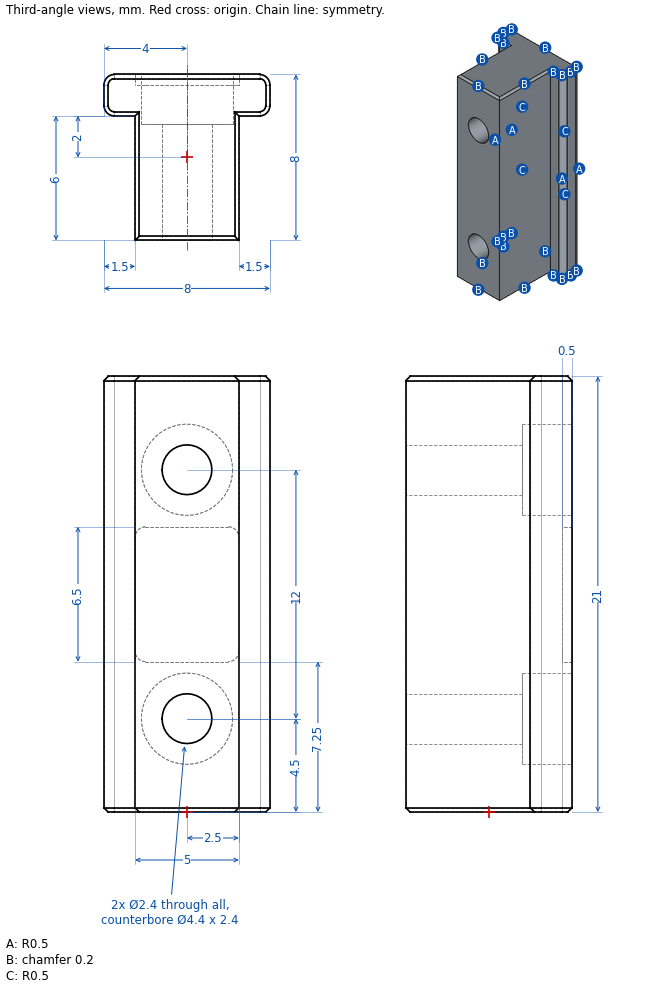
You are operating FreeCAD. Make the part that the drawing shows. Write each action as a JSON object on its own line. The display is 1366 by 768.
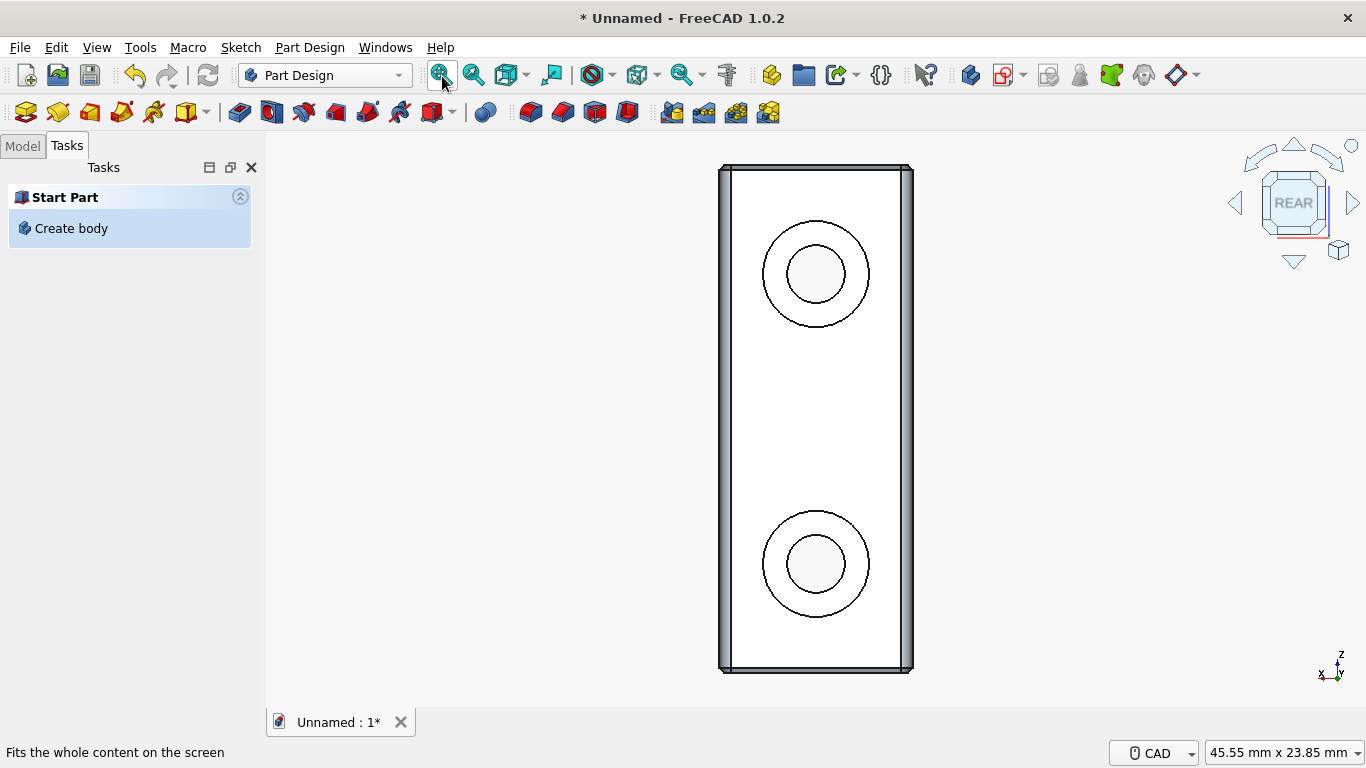
{"action": "left_click", "coordinate": [816, 418]}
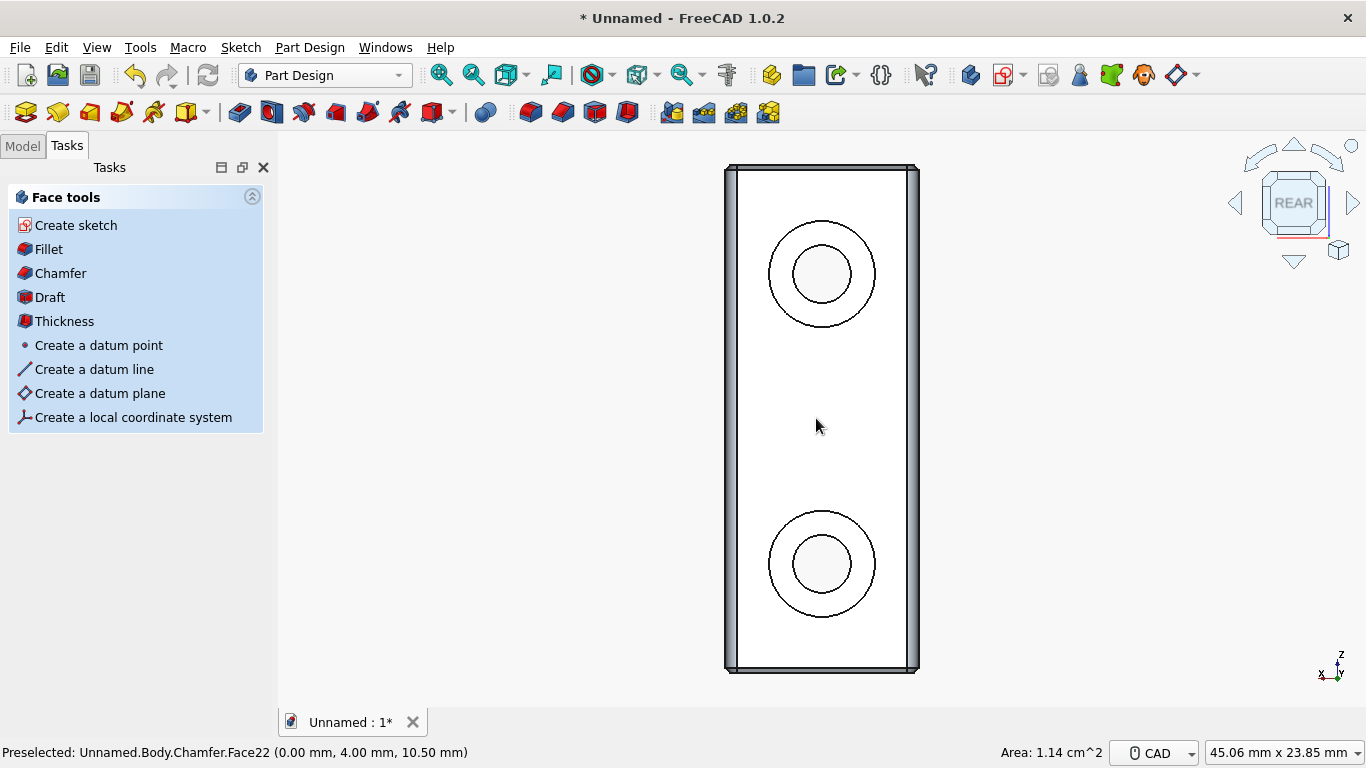
{"action": "left_click", "coordinate": [1004, 76]}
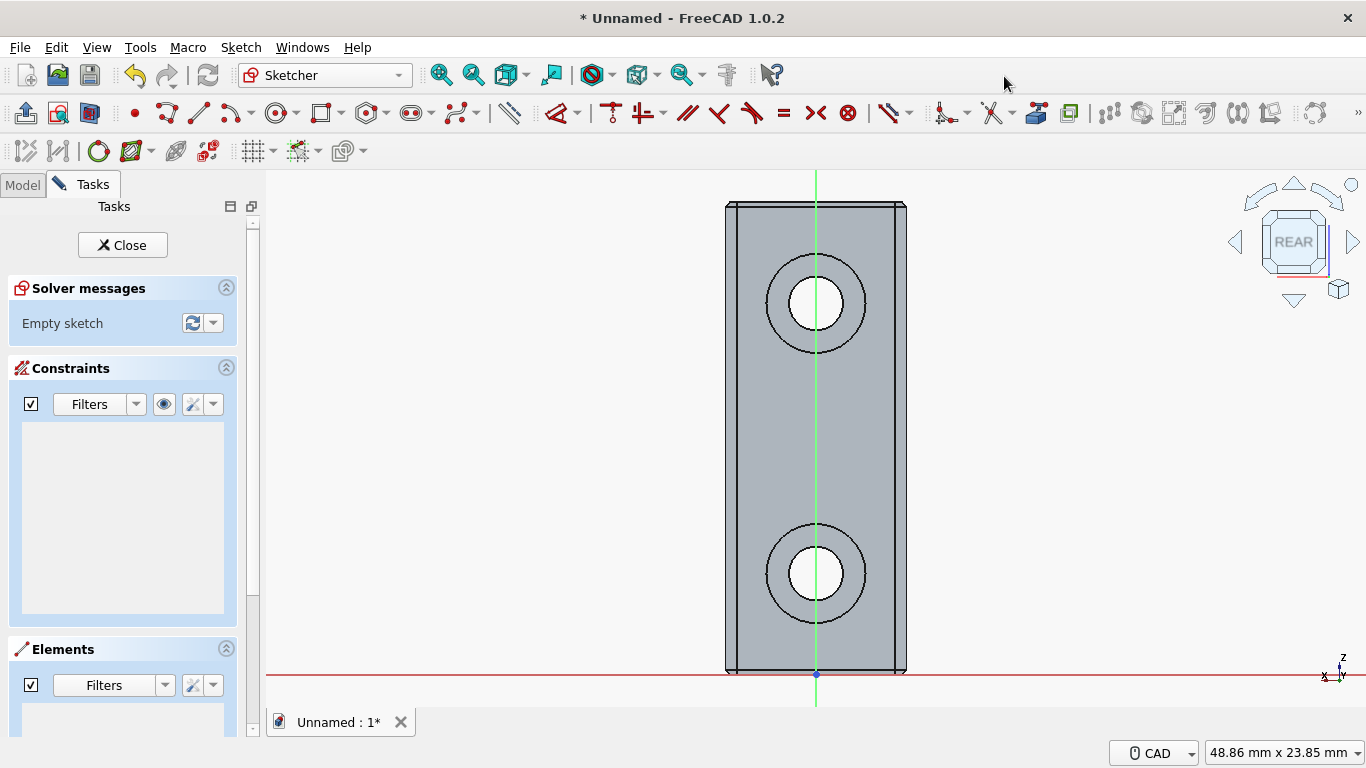
{"action": "scroll", "coordinate": [438, 198], "scroll_direction": "down", "scroll_amount": 1}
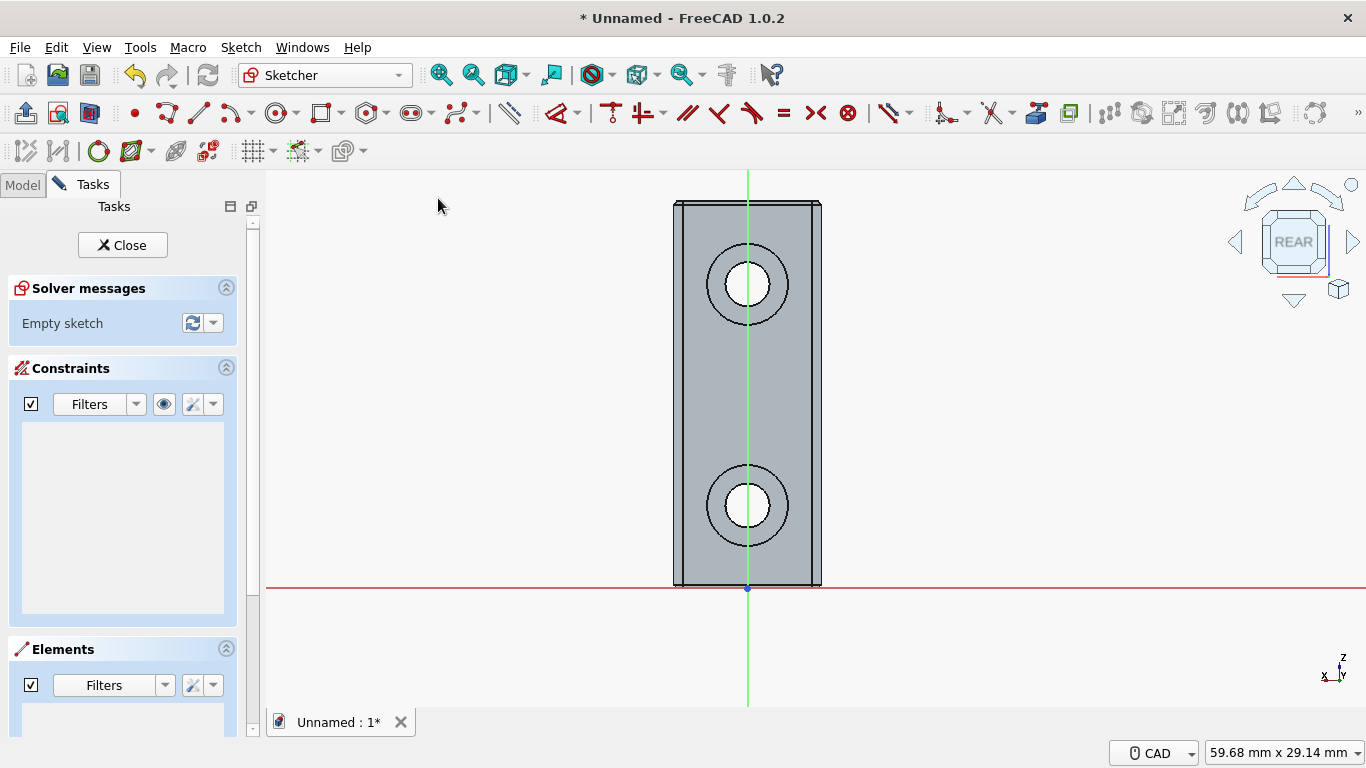
{"action": "left_click", "coordinate": [322, 114]}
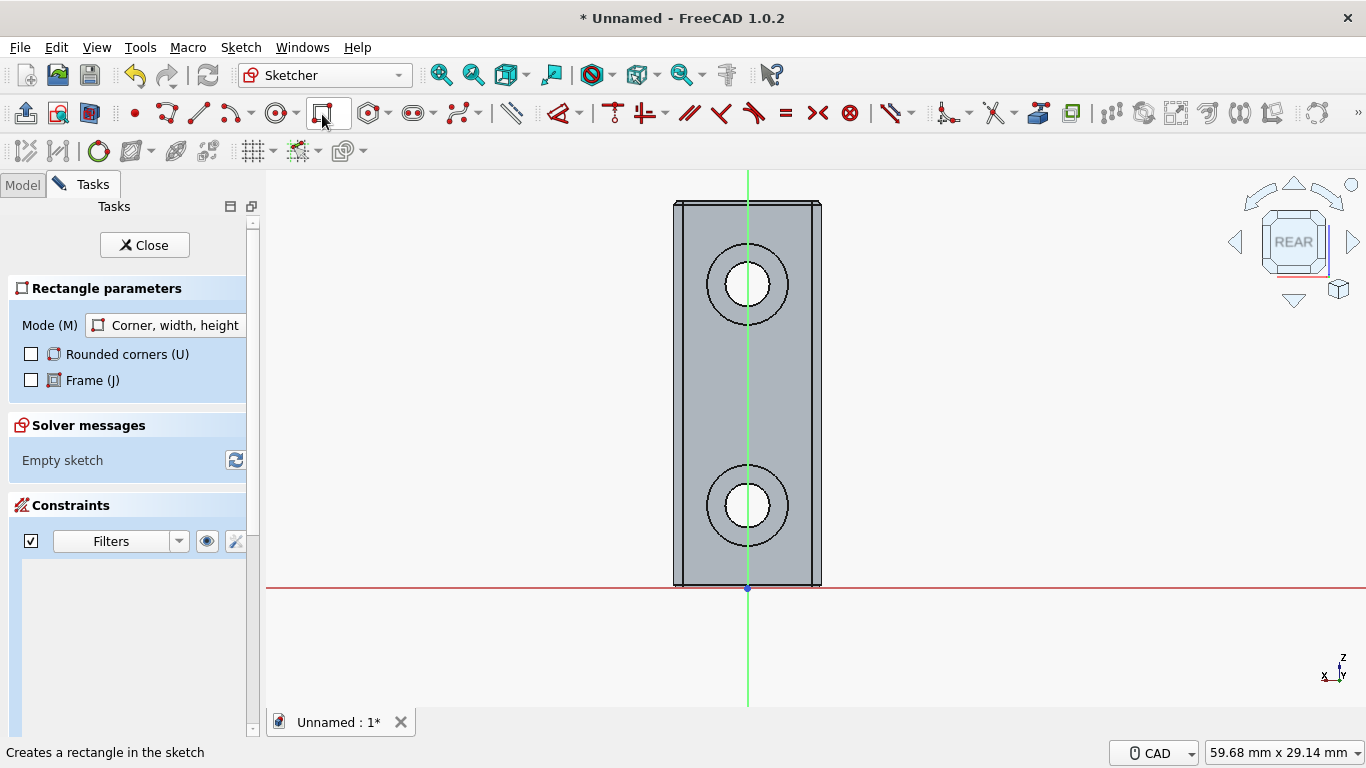
{"action": "left_click", "coordinate": [701, 335]}
{"action": "mouse_move", "coordinate": [794, 455]}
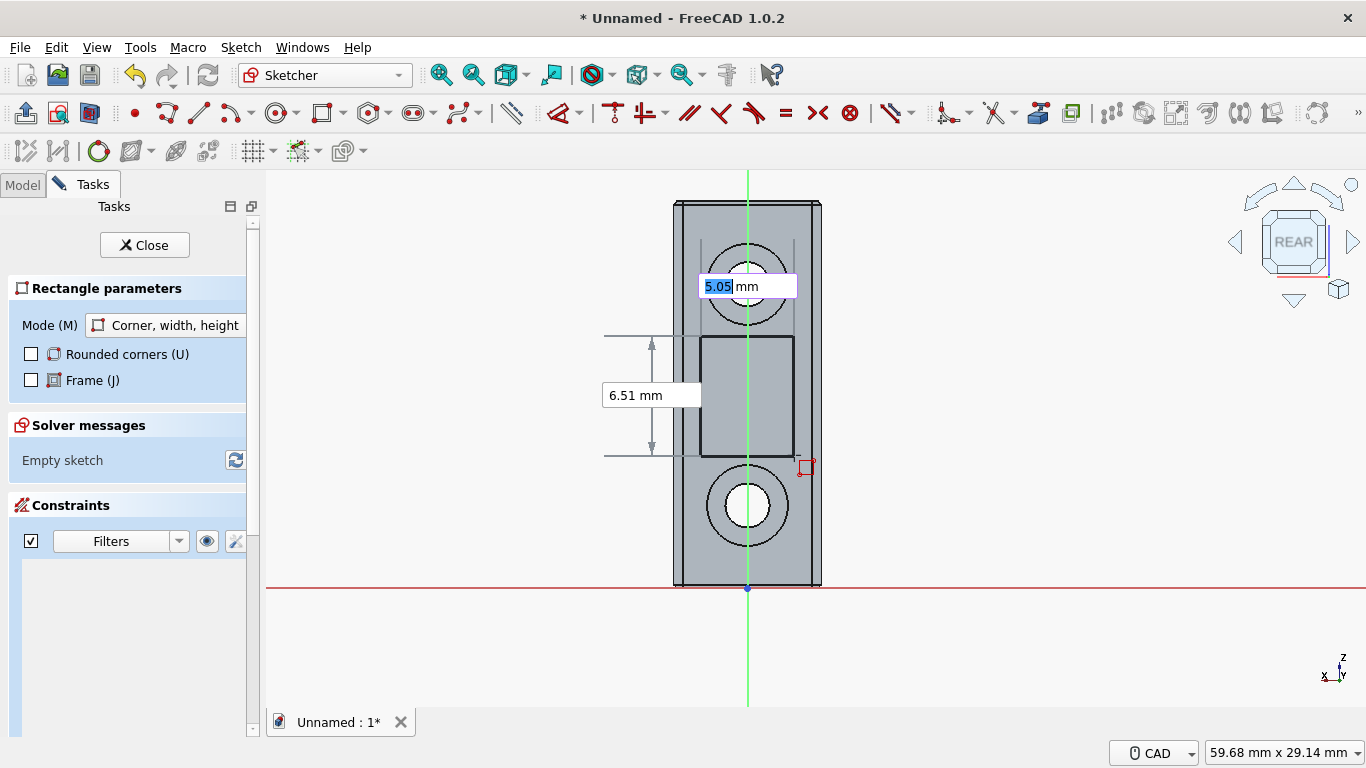
{"action": "type", "text": "5"}
{"action": "key", "text": "Tab"}
{"action": "type", "text": "6.5"}
{"action": "key", "text": "Return"}
{"action": "key", "text": "Escape"}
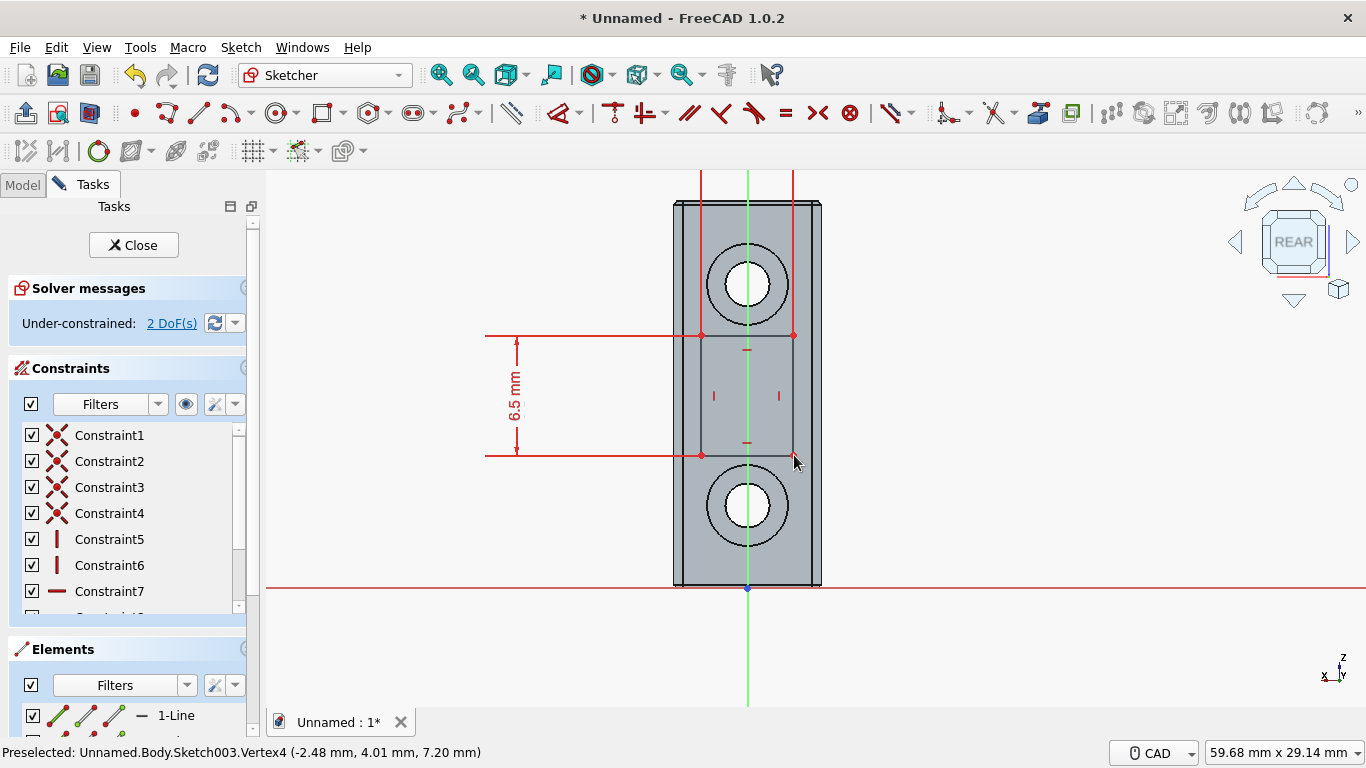
{"action": "left_click", "coordinate": [558, 114]}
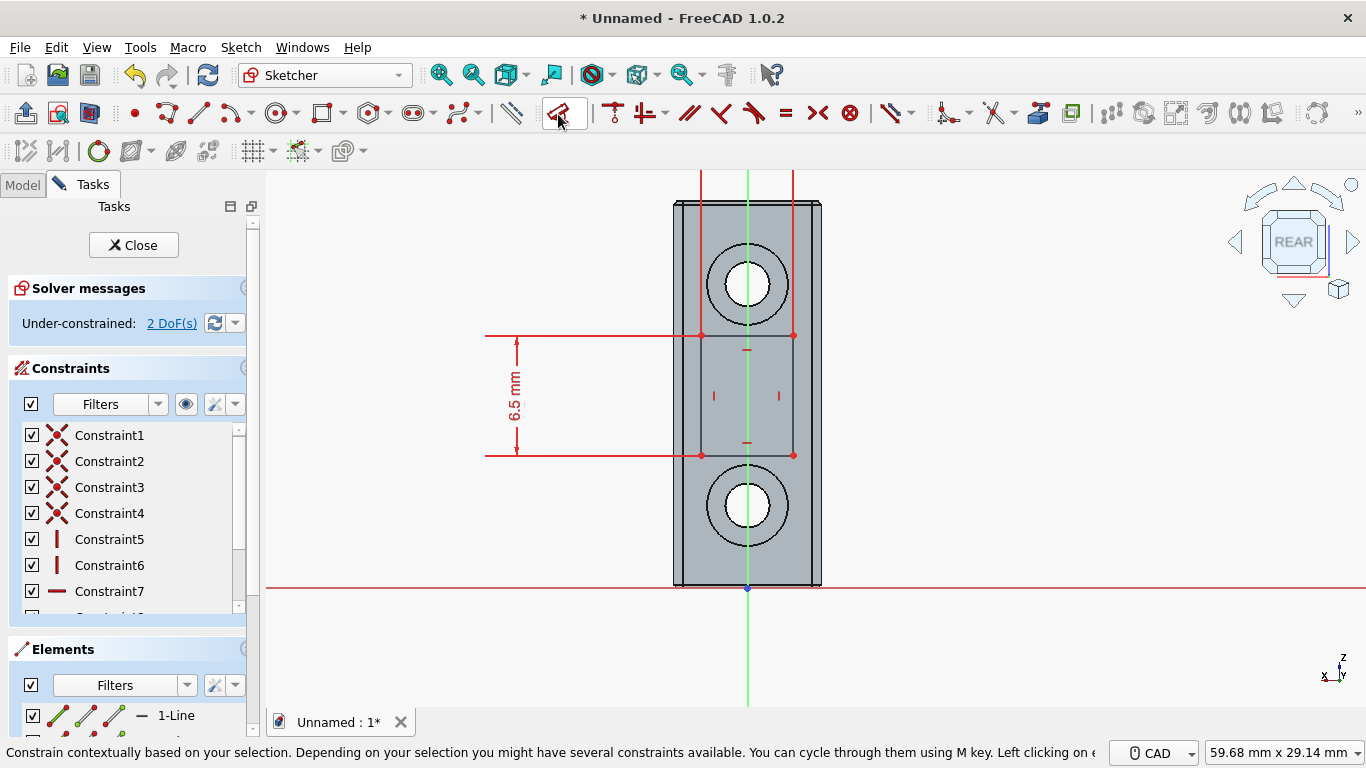
{"action": "left_click", "coordinate": [701, 336]}
{"action": "left_click", "coordinate": [724, 622]}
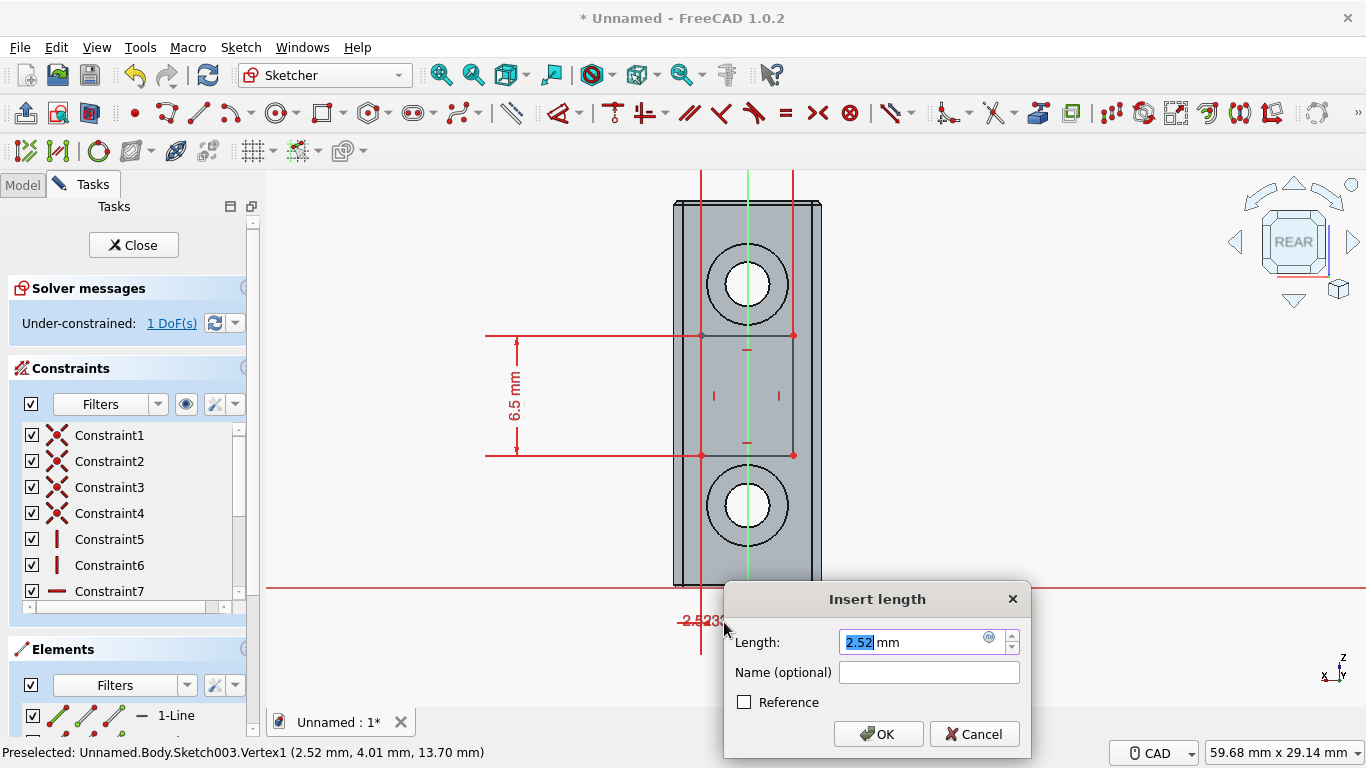
{"action": "type", "text": "2.5"}
{"action": "key", "text": "Return"}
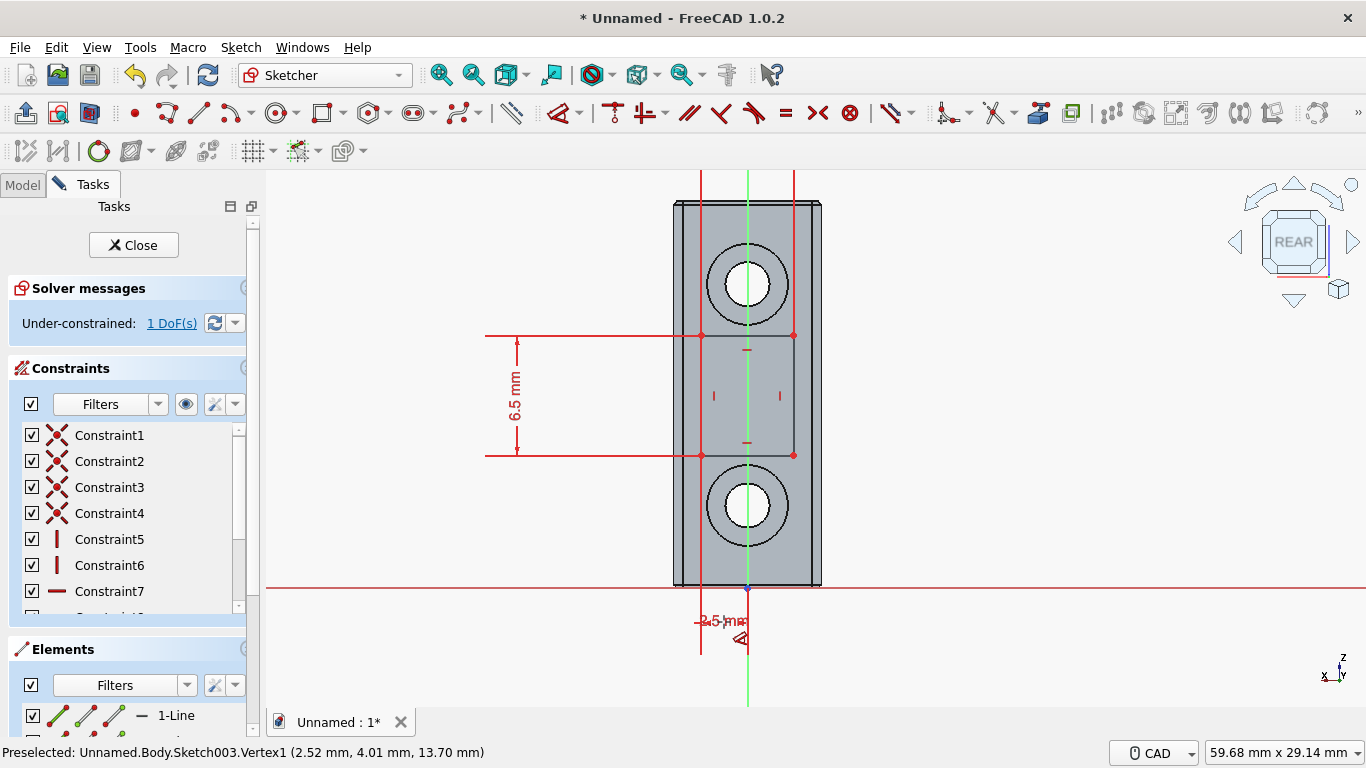
{"action": "left_click", "coordinate": [701, 456]}
{"action": "left_click", "coordinate": [667, 522]}